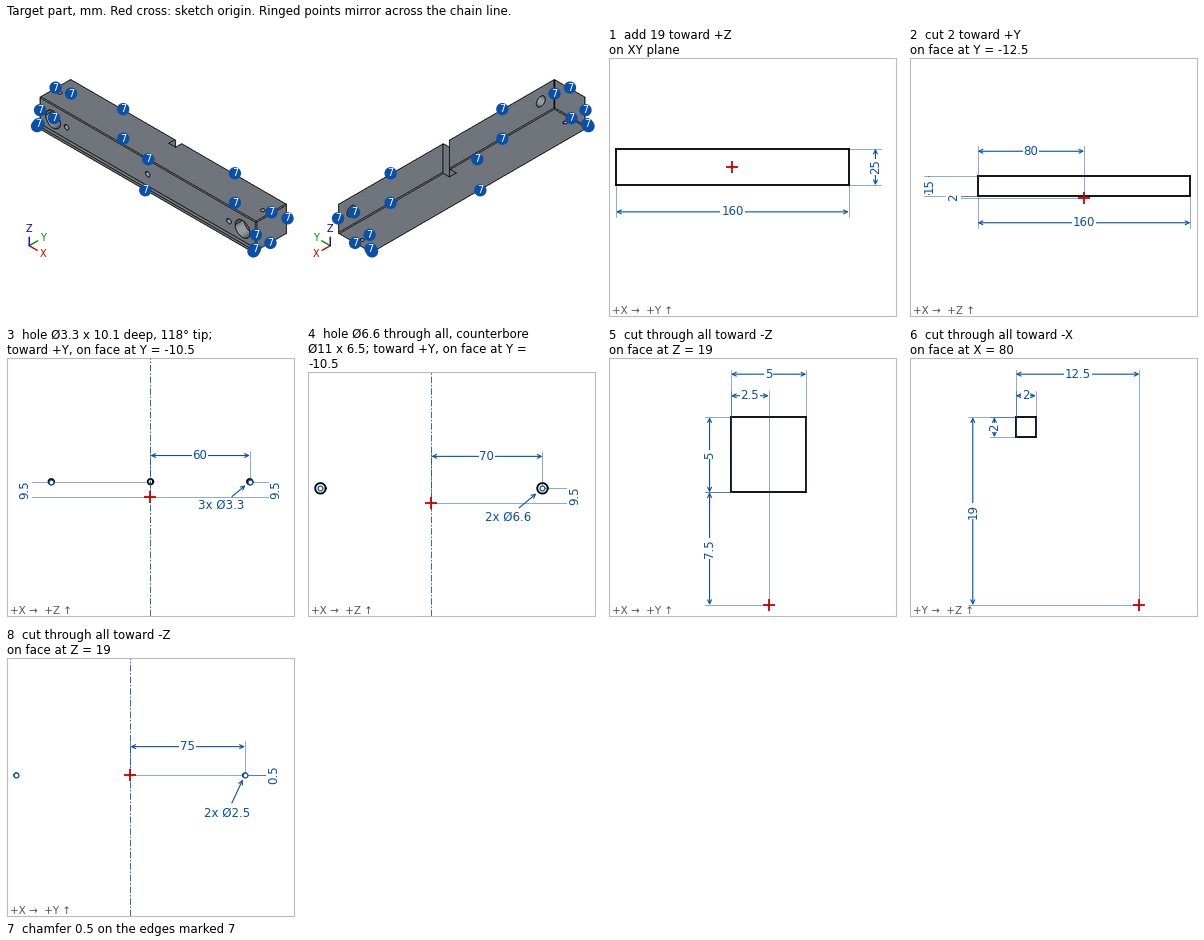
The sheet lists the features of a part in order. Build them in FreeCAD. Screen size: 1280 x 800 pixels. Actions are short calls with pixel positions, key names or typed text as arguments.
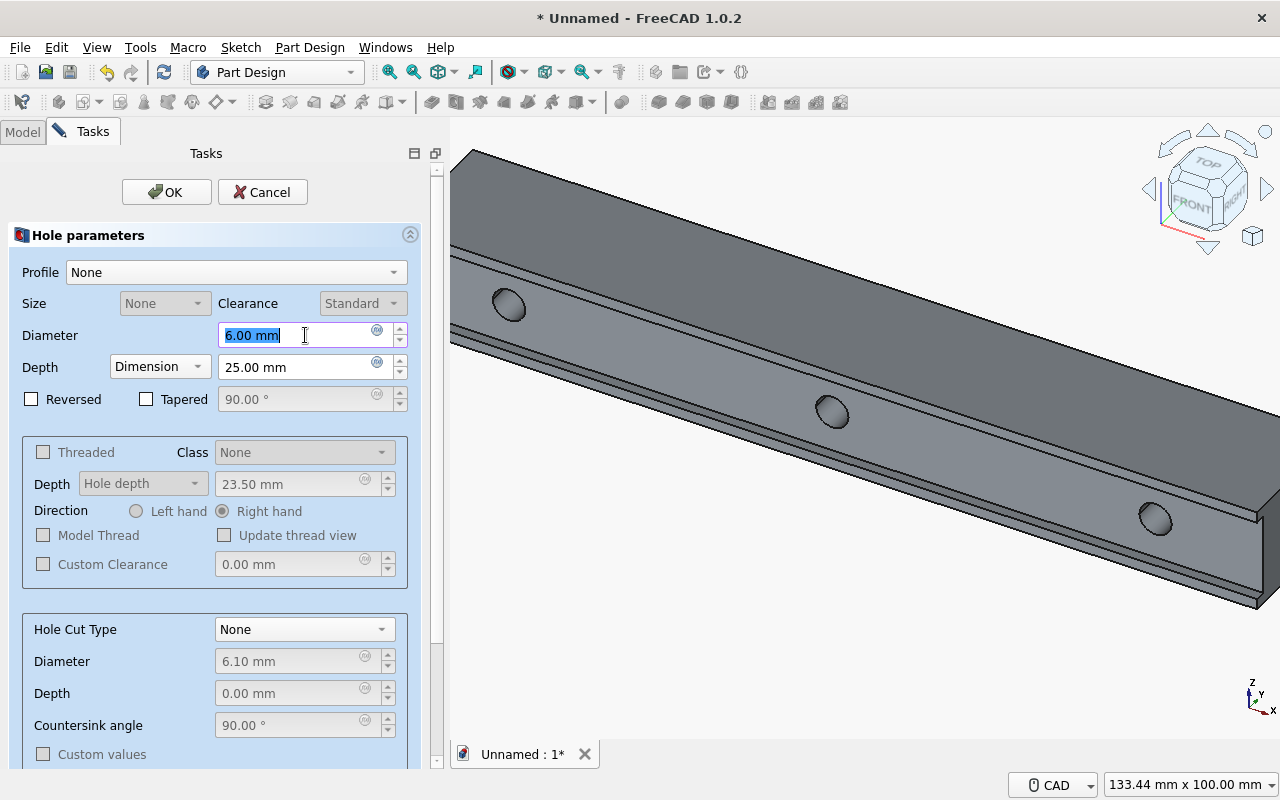
text(3.3)
key(Tab)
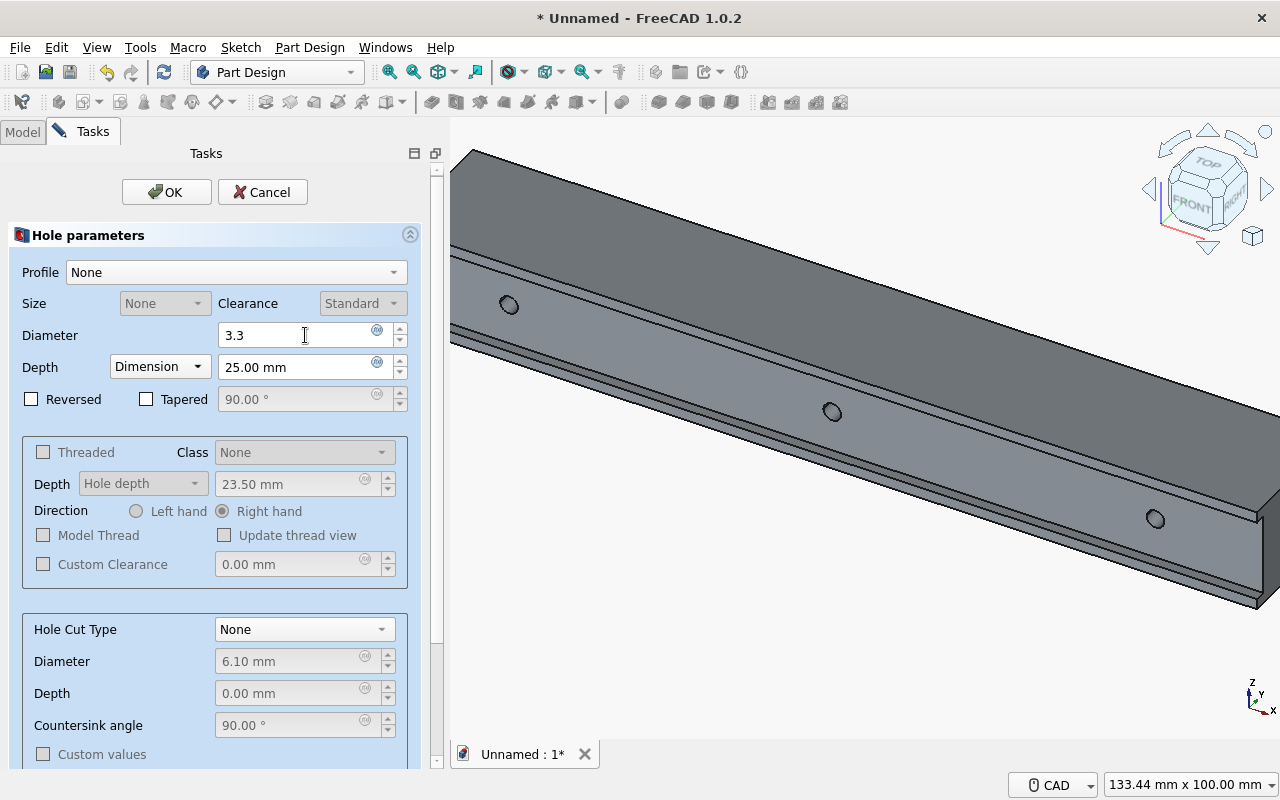
triple_click(305, 367)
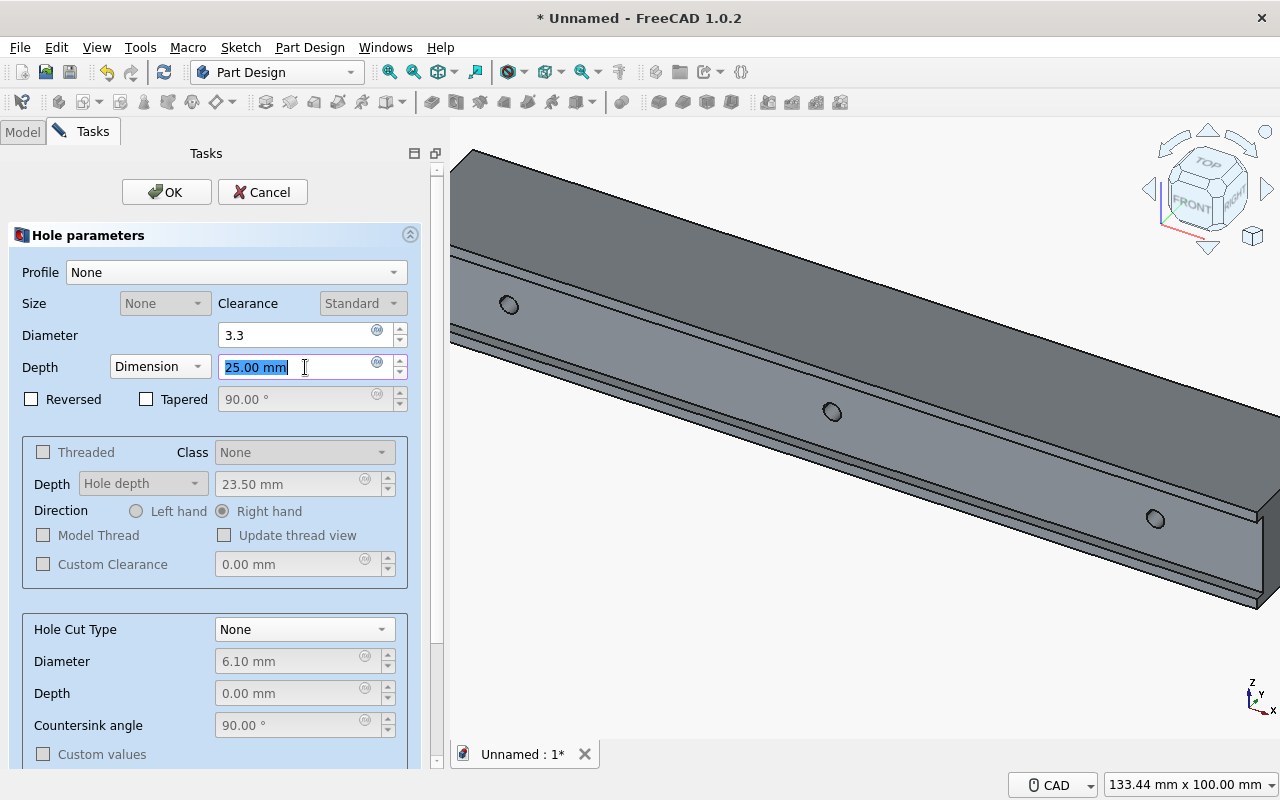
text(10.1)
key(Tab)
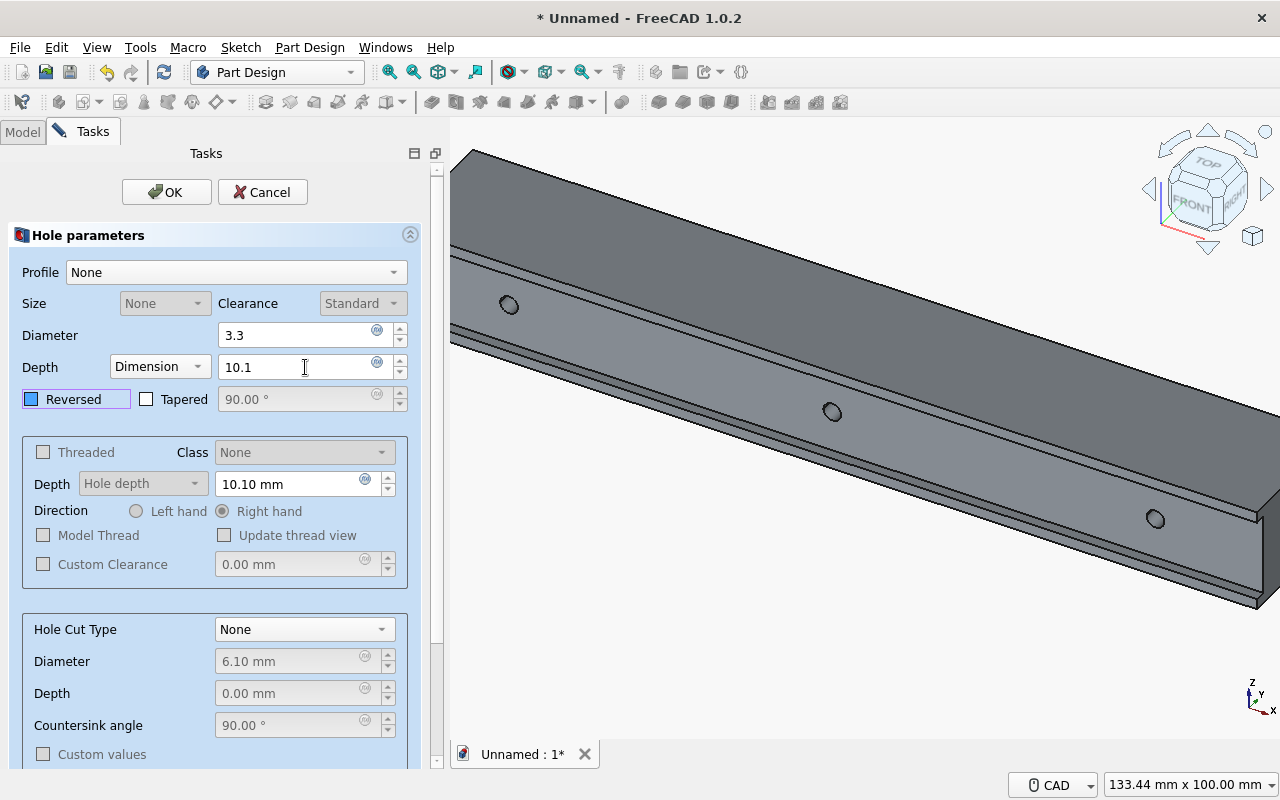
click(167, 192)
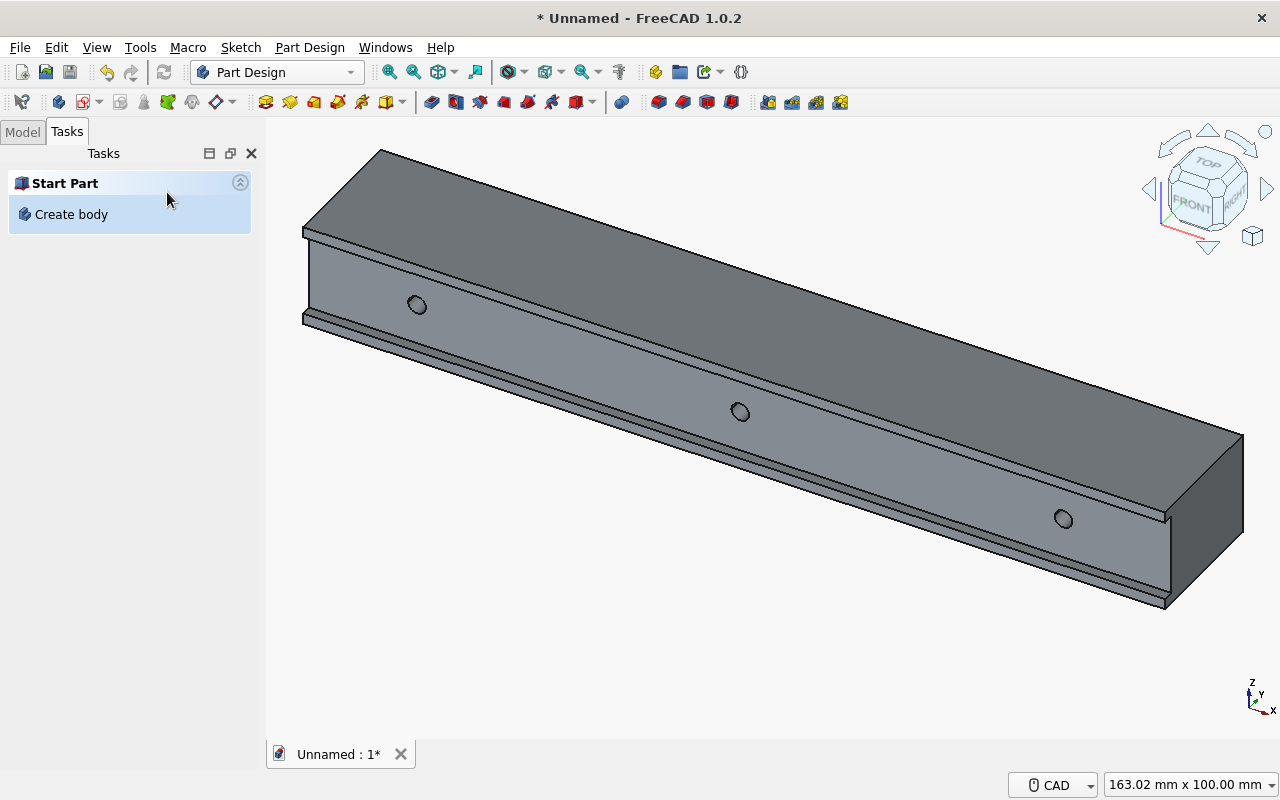
click(987, 493)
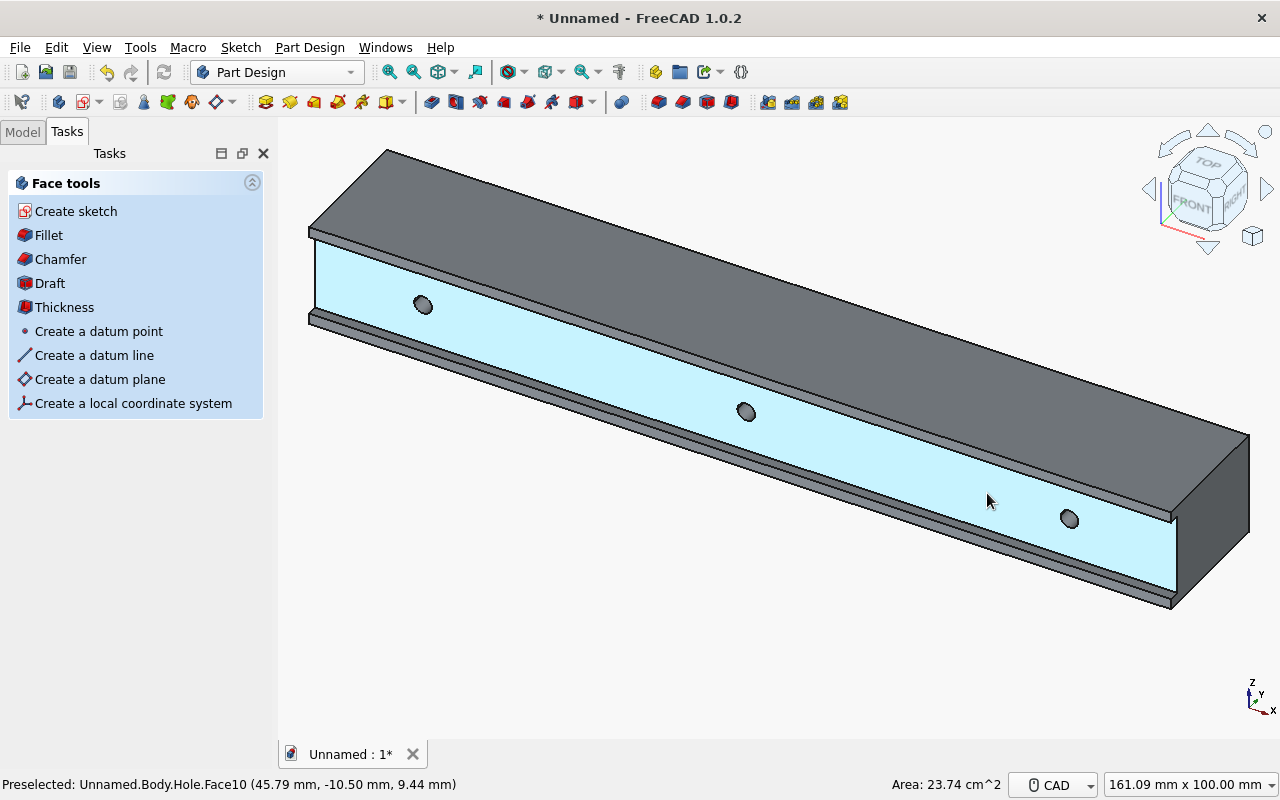
click(84, 102)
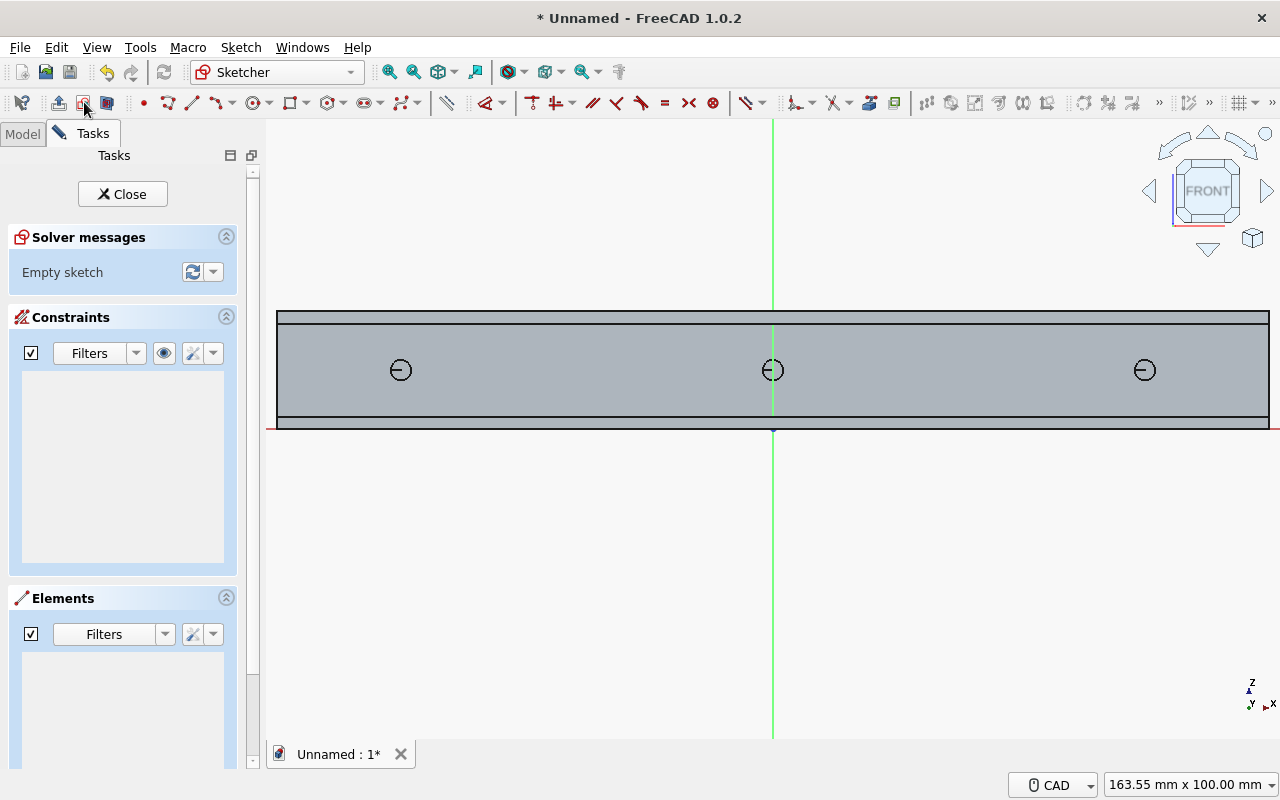
scroll(565, 510, down, 2)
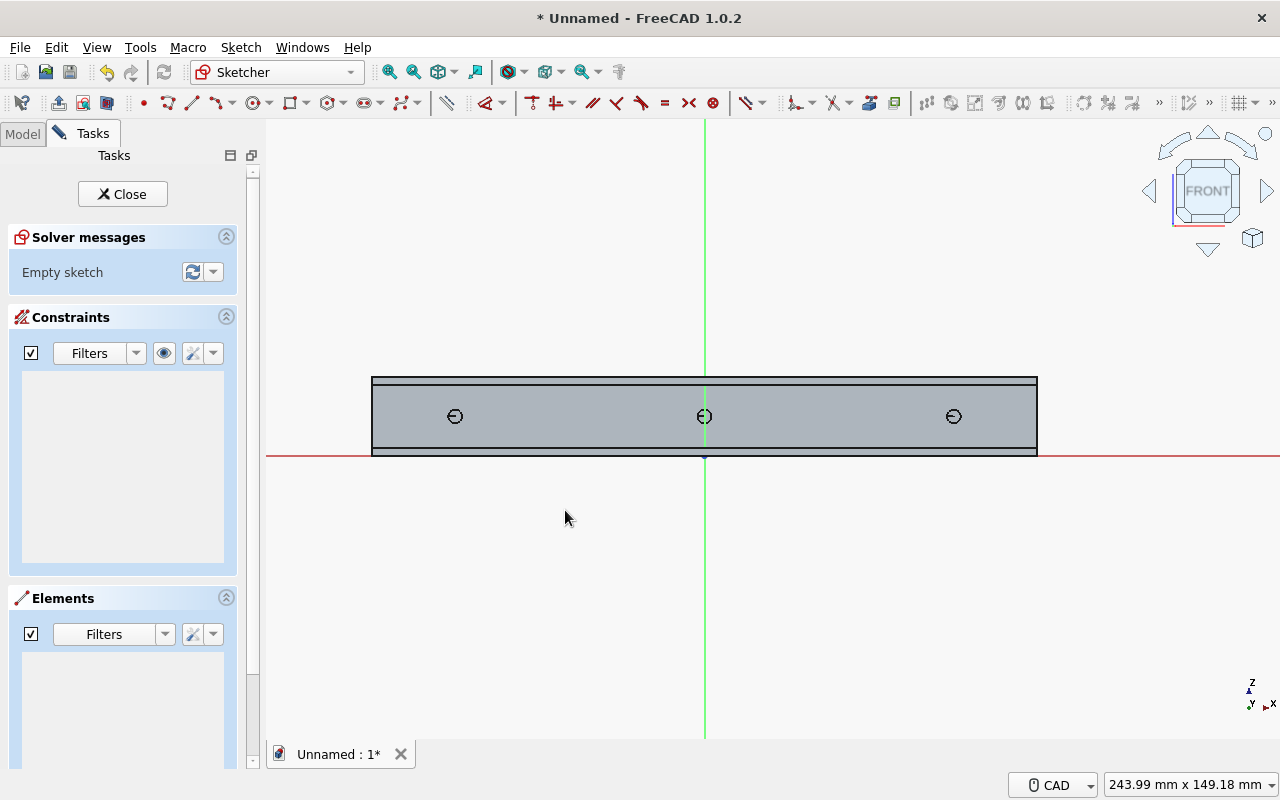
click(254, 104)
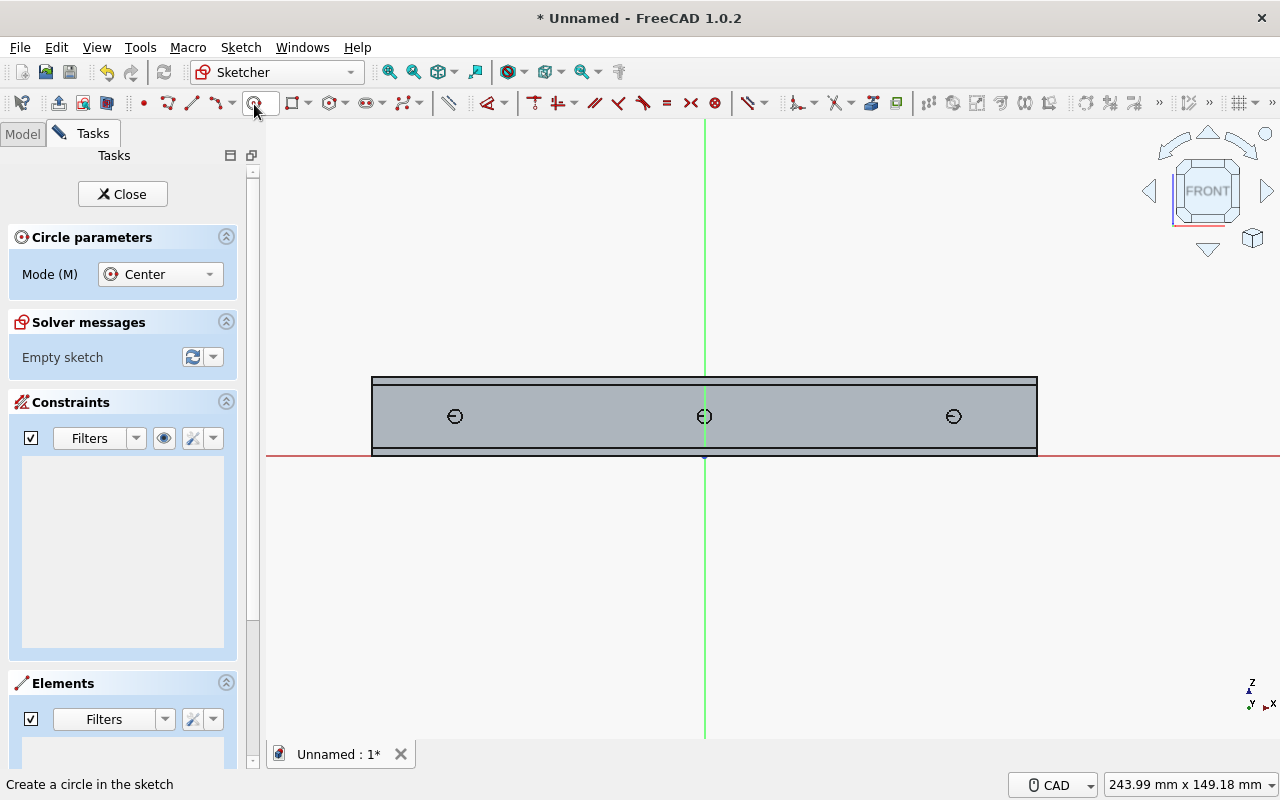
scroll(995, 416, up, 3)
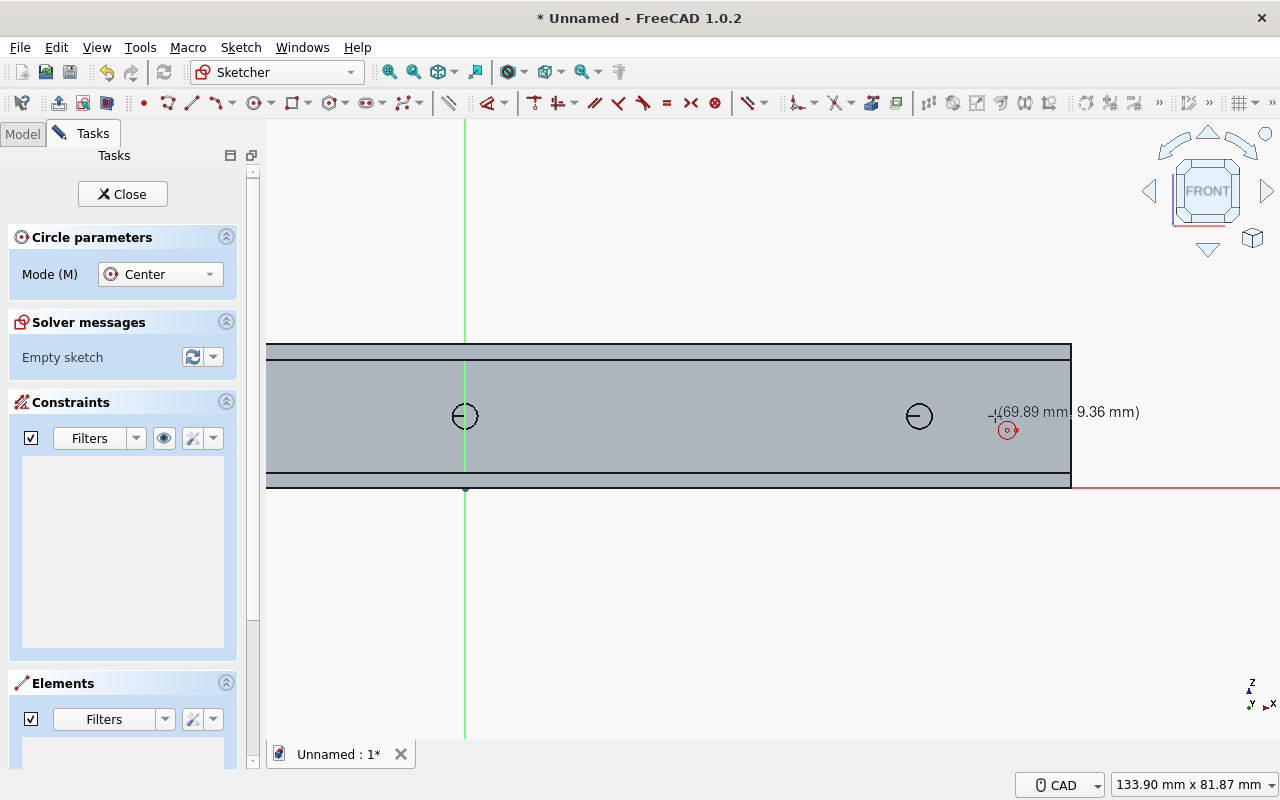
click(995, 416)
click(1013, 399)